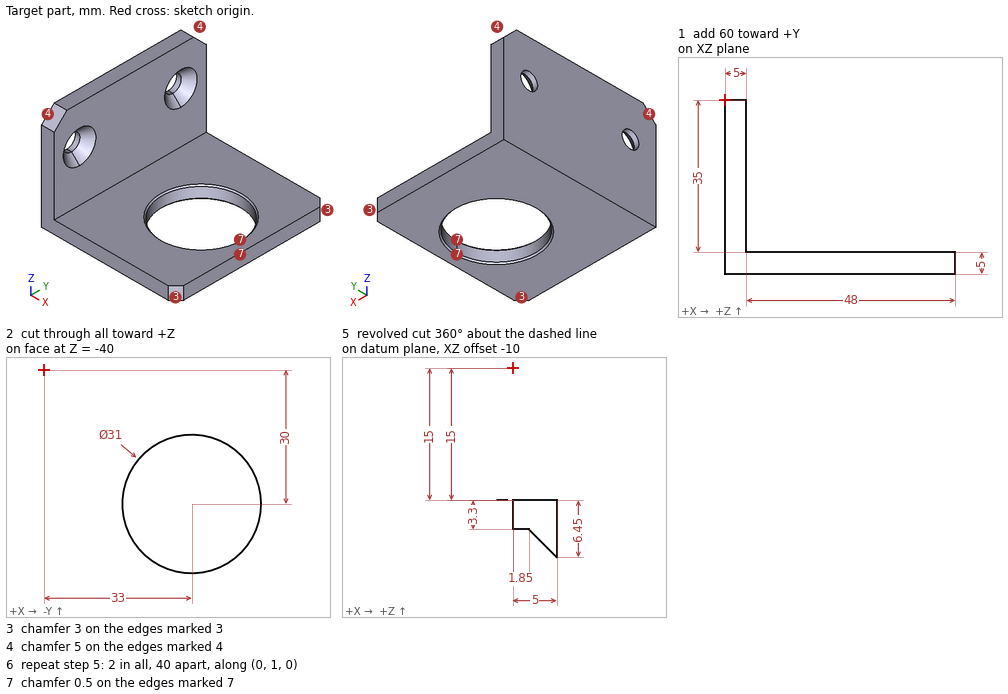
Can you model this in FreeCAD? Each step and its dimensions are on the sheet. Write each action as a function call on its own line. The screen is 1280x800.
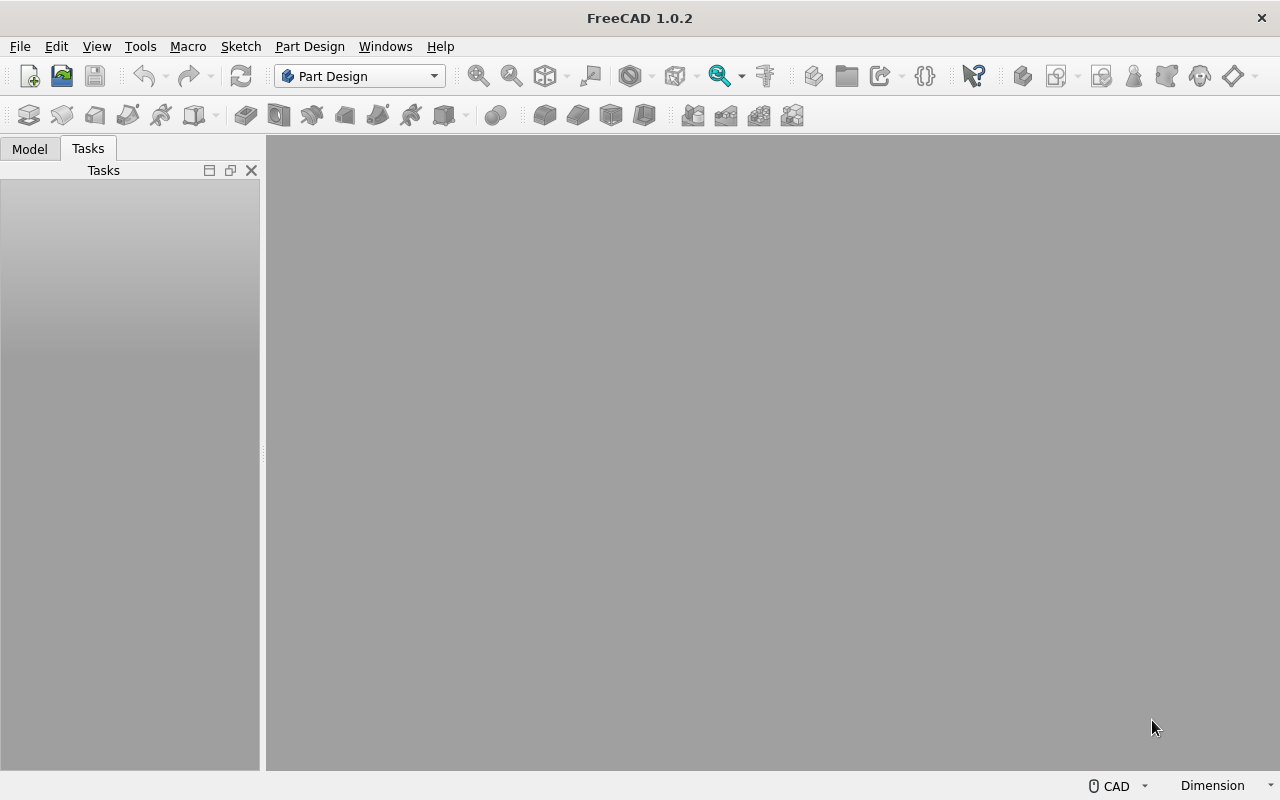
click(29, 76)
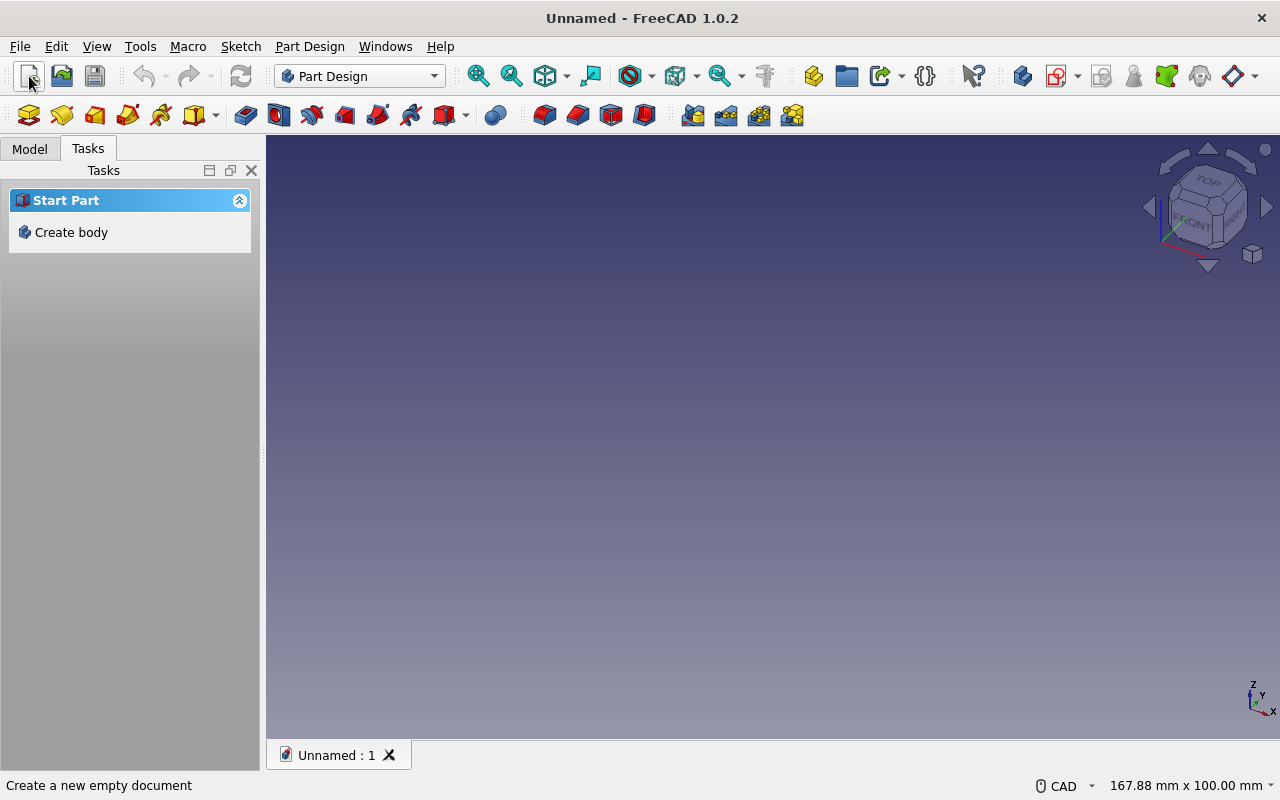
click(1056, 76)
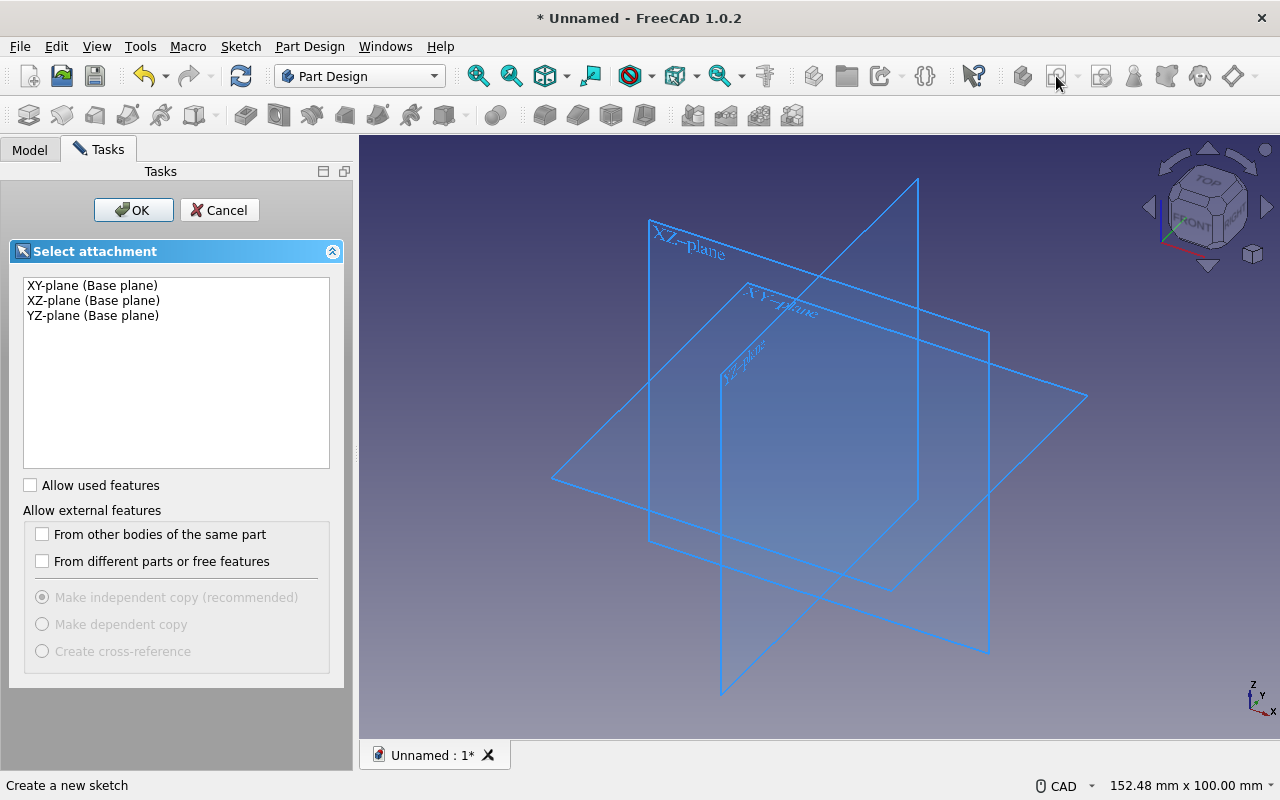
click(84, 300)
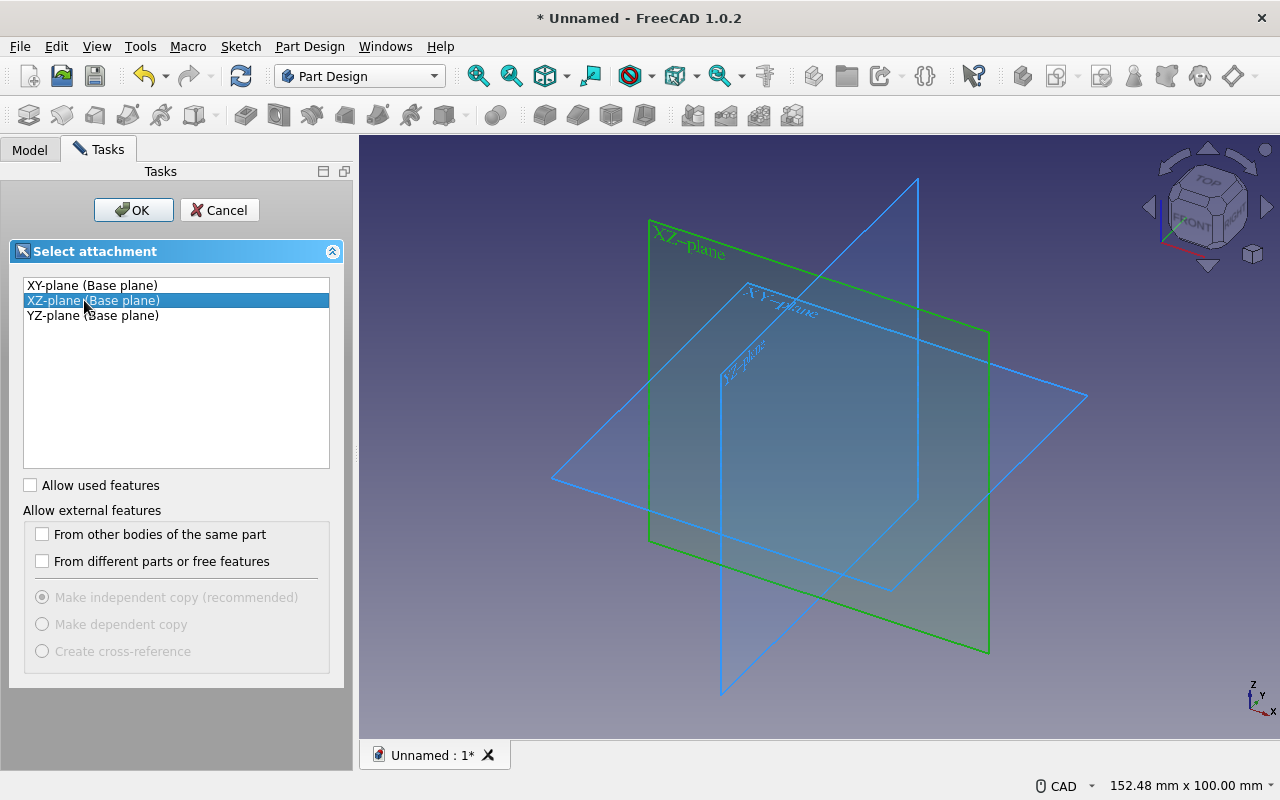
click(134, 210)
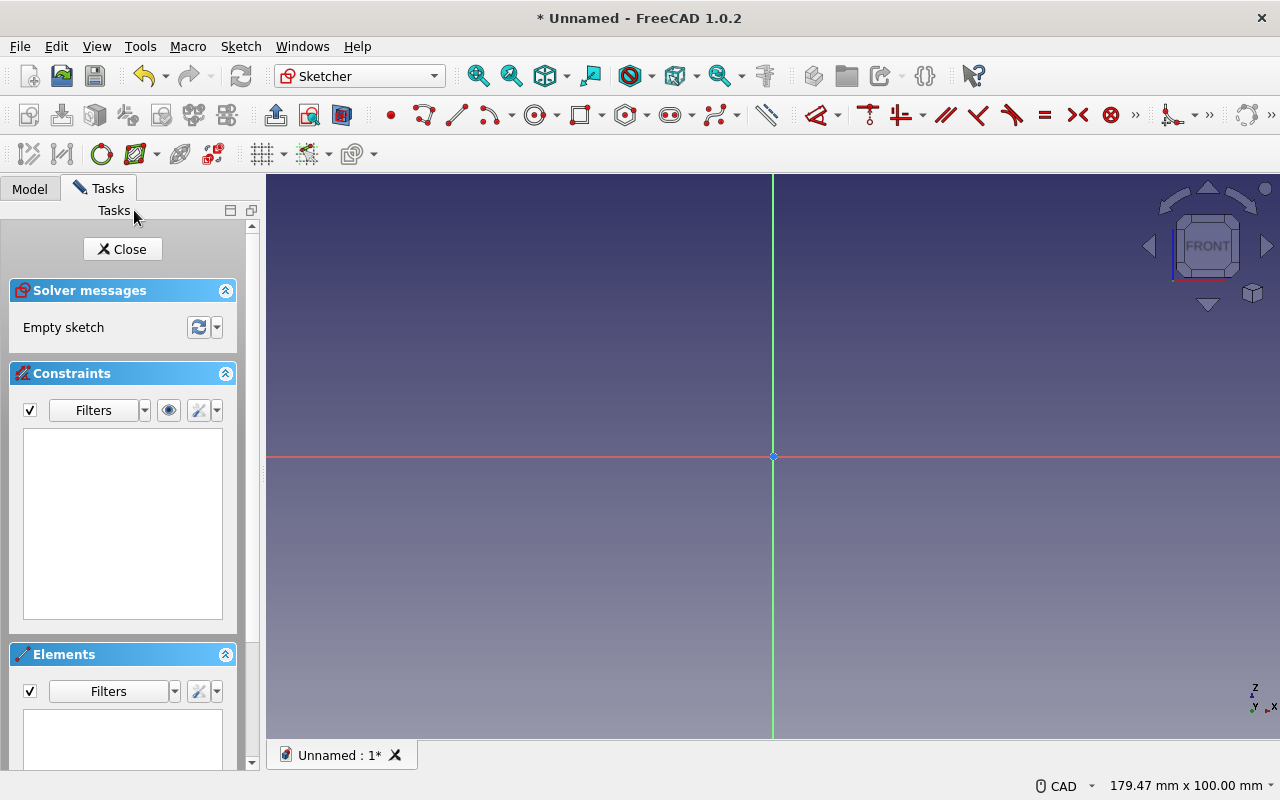
scroll(1115, 711, up, 2)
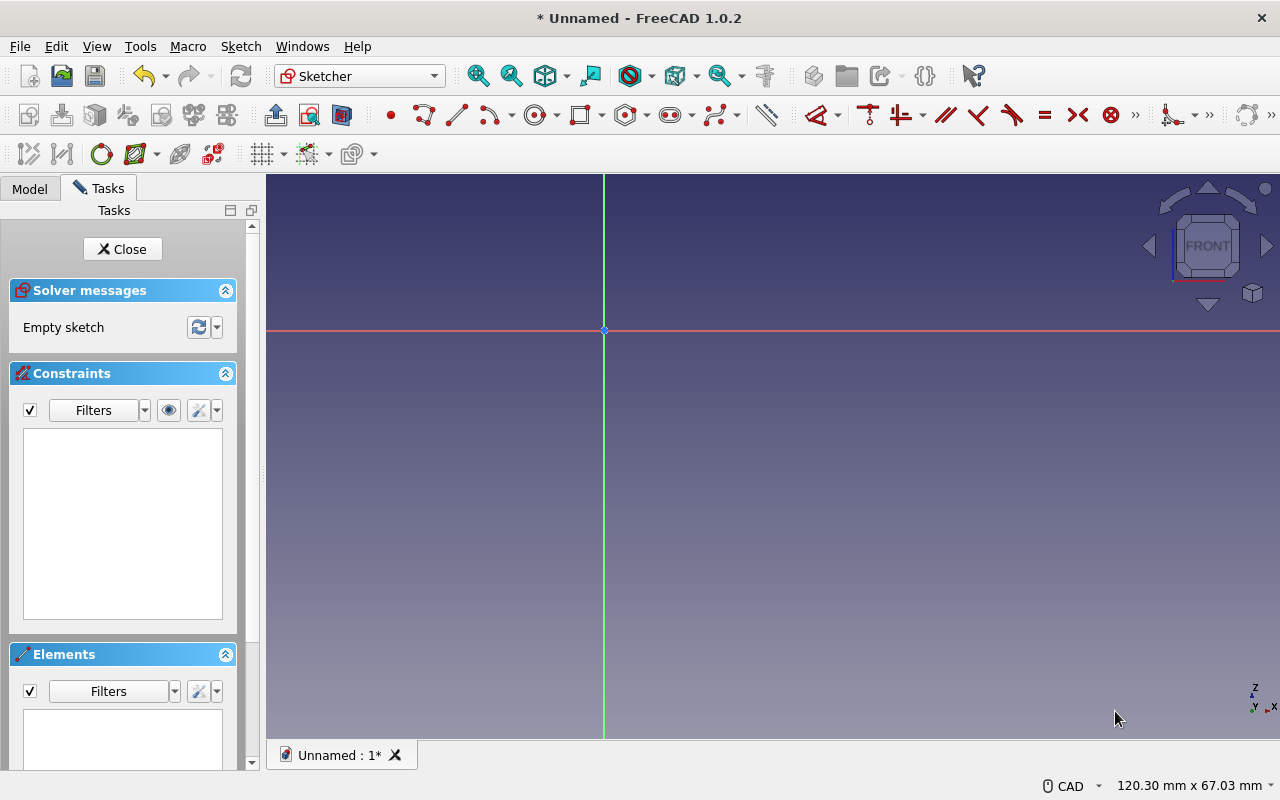
key(g)
key(m)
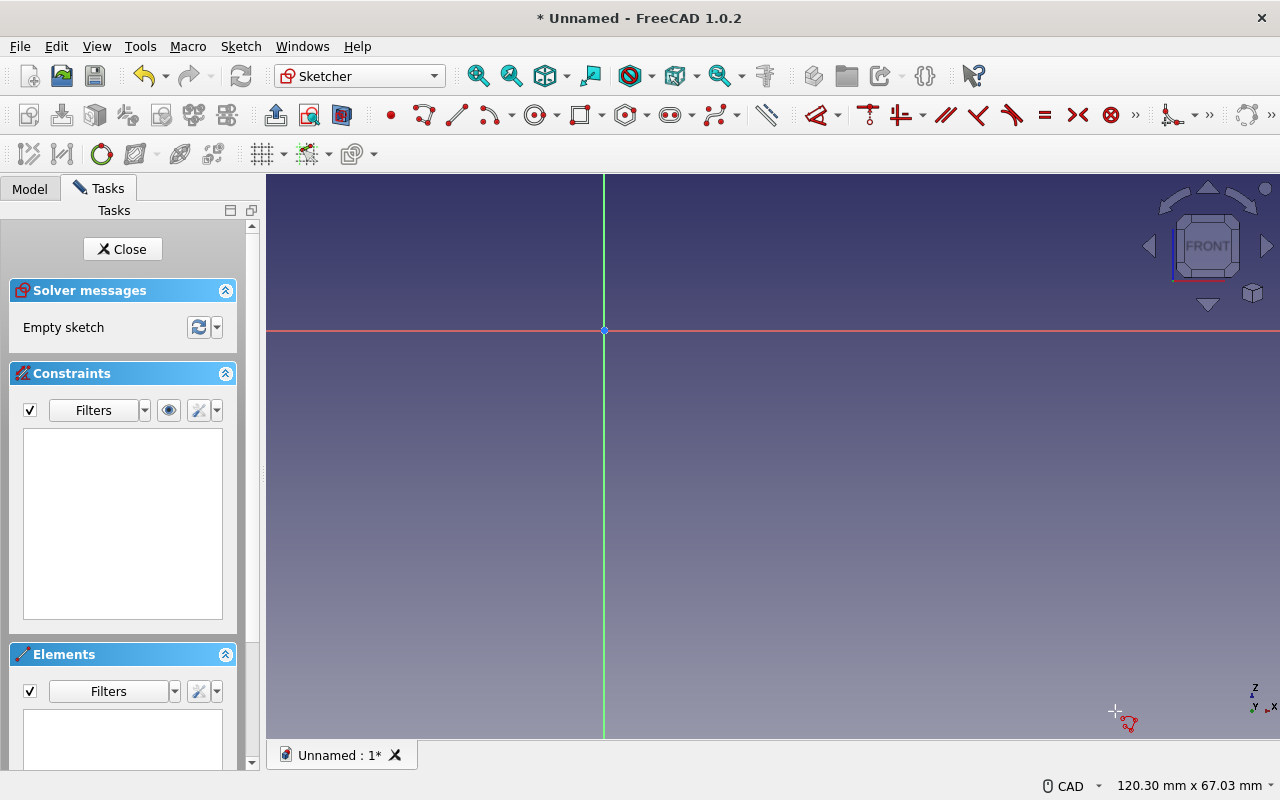
click(604, 331)
click(647, 340)
click(647, 626)
click(1051, 626)
click(1051, 668)
click(613, 668)
click(604, 331)
key(Escape)
key(Escape)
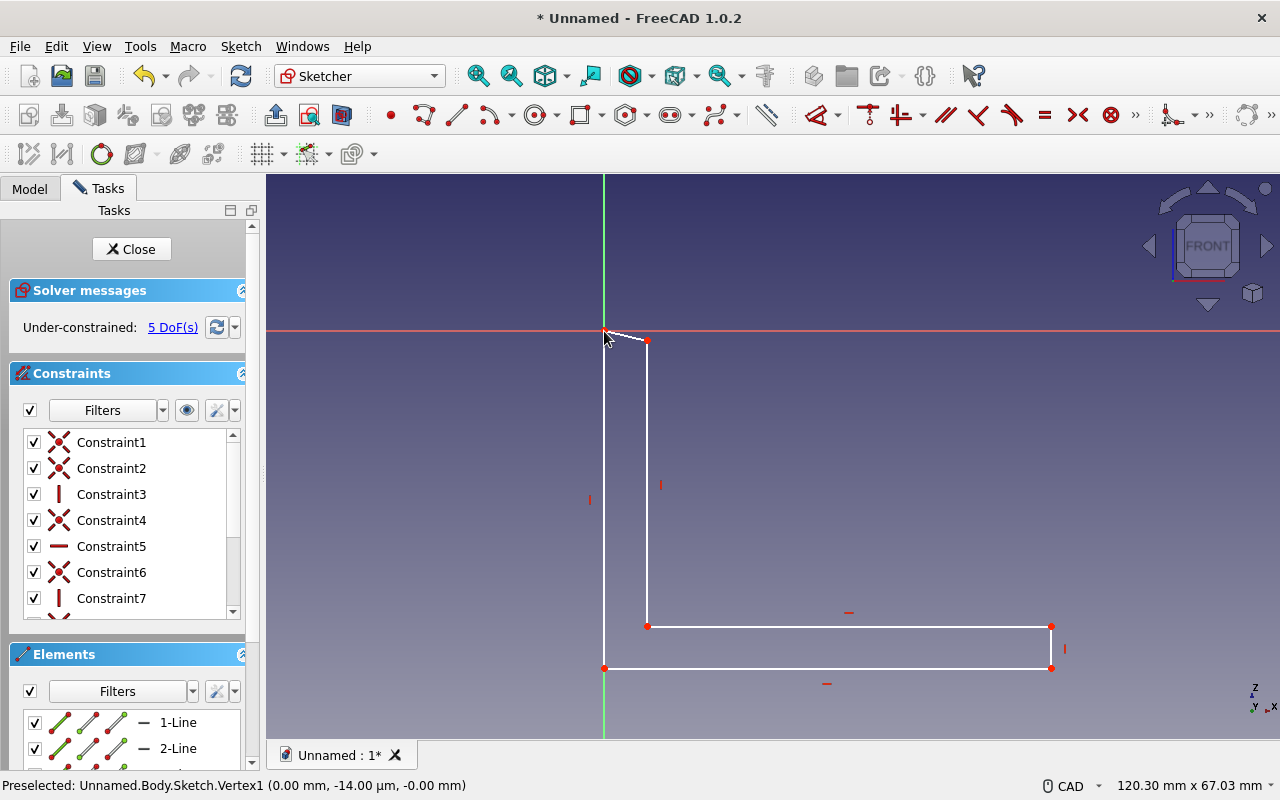
click(617, 334)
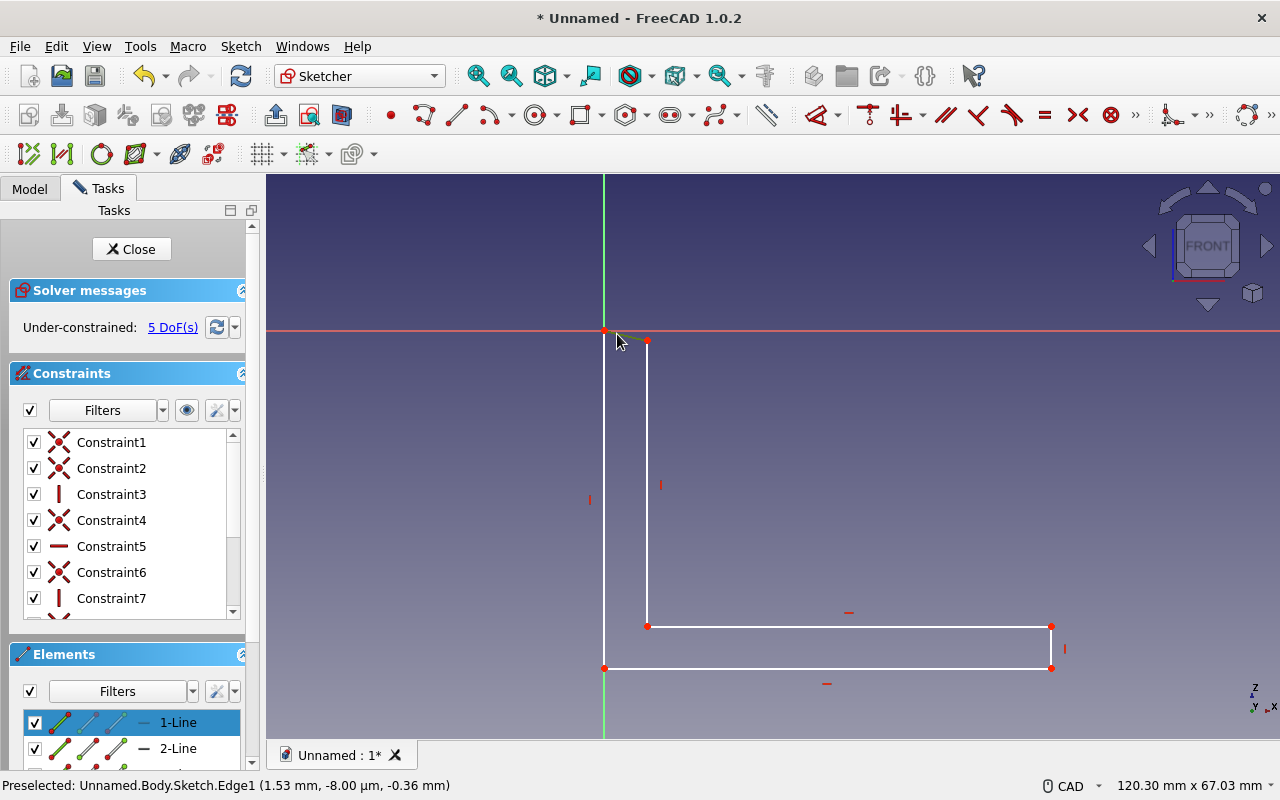
key(h)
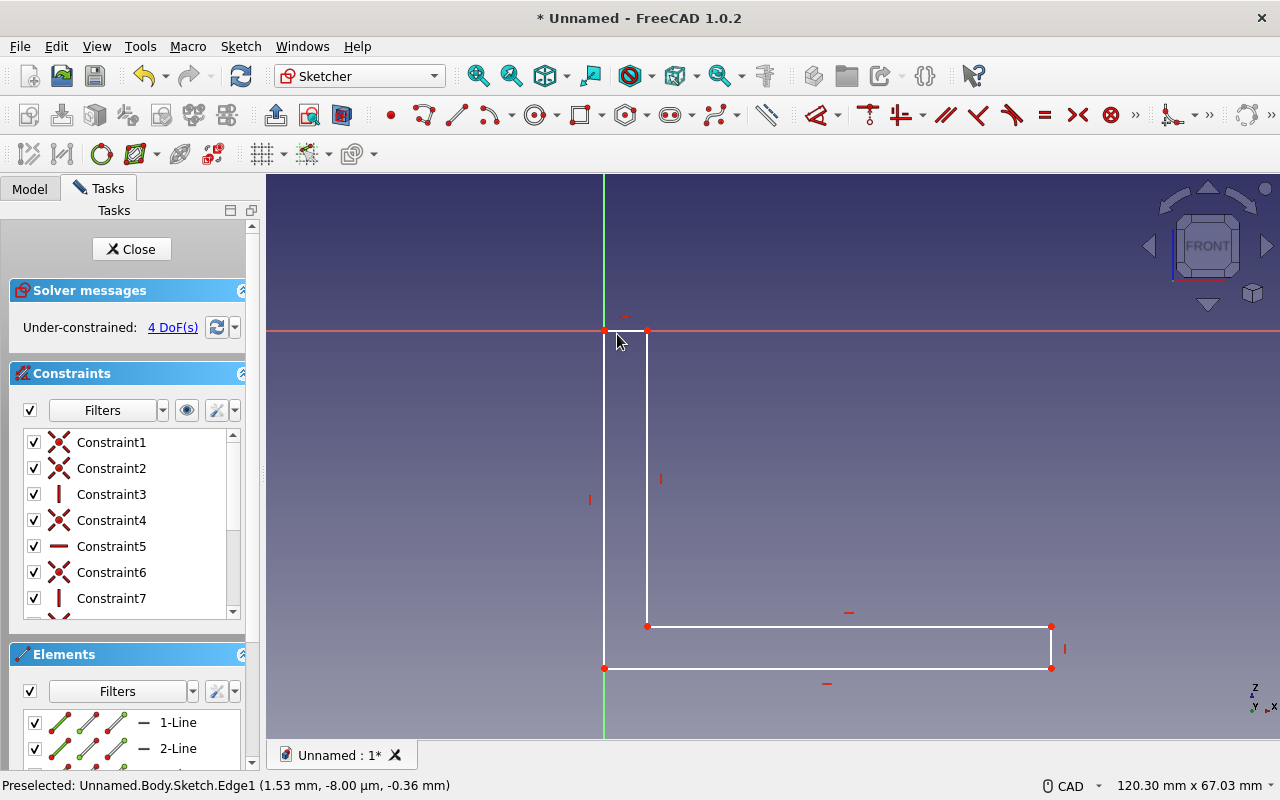
click(617, 331)